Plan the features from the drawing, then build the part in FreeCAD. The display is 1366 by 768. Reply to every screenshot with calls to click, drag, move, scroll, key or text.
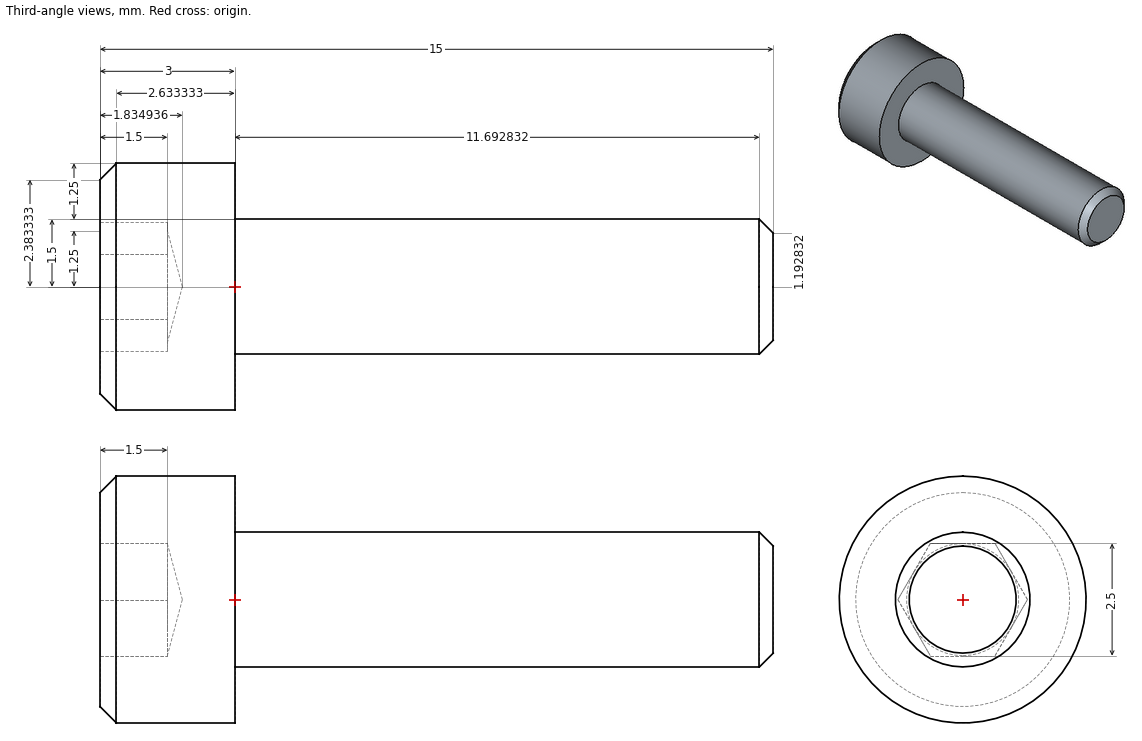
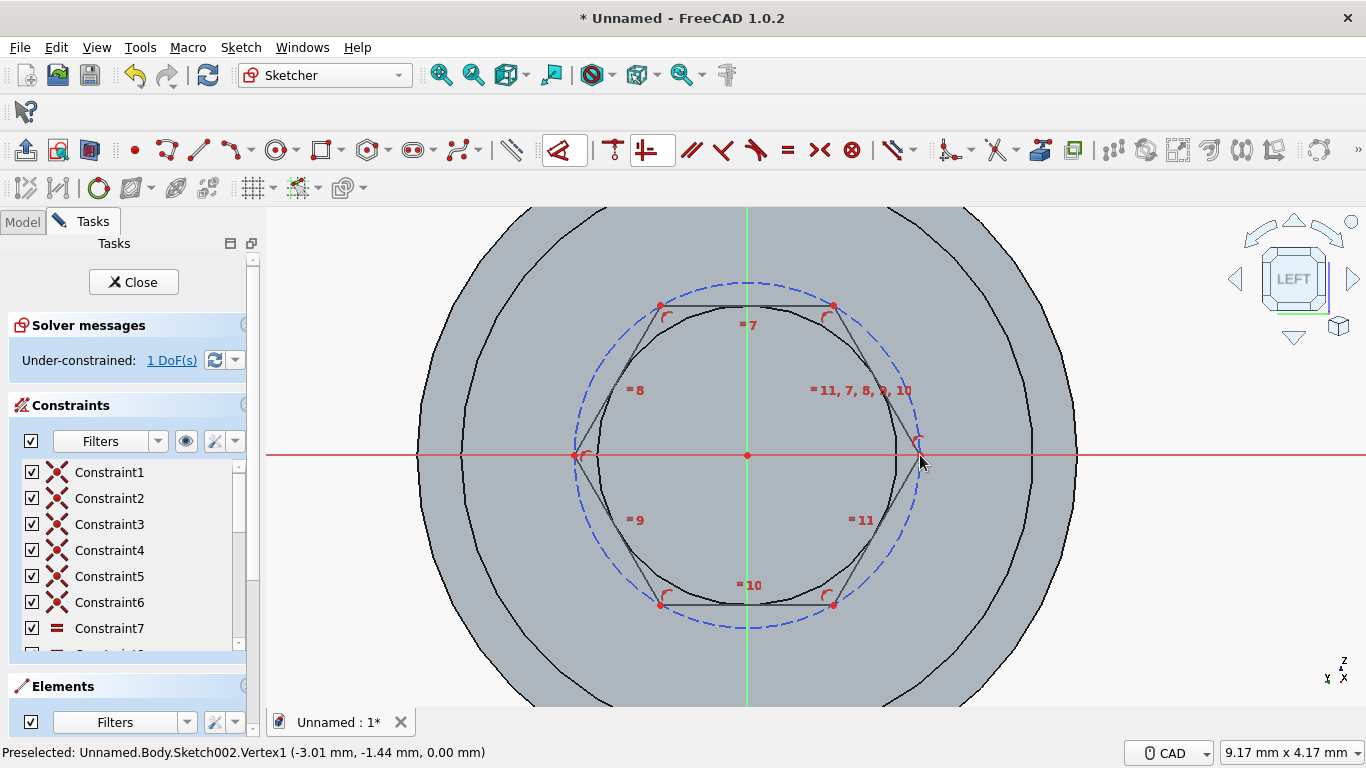
click(661, 605)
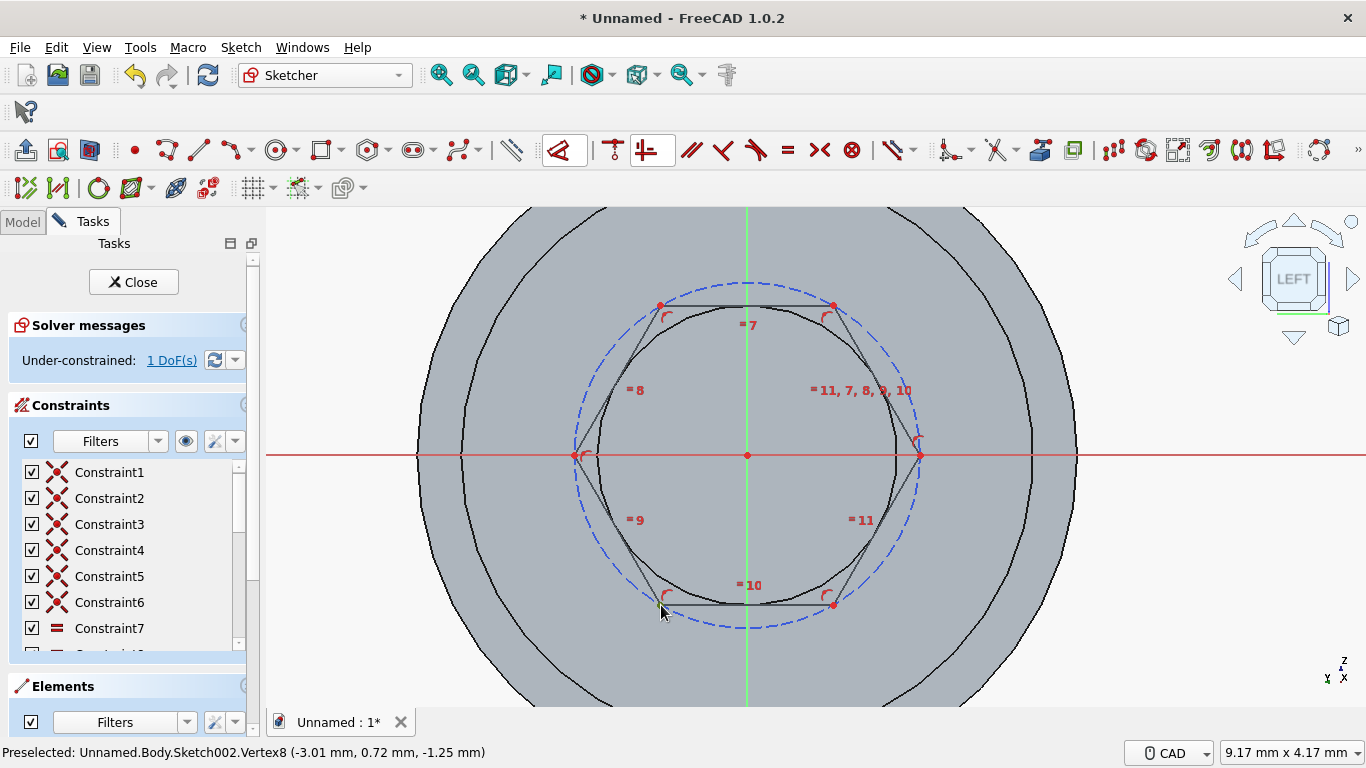
click(834, 306)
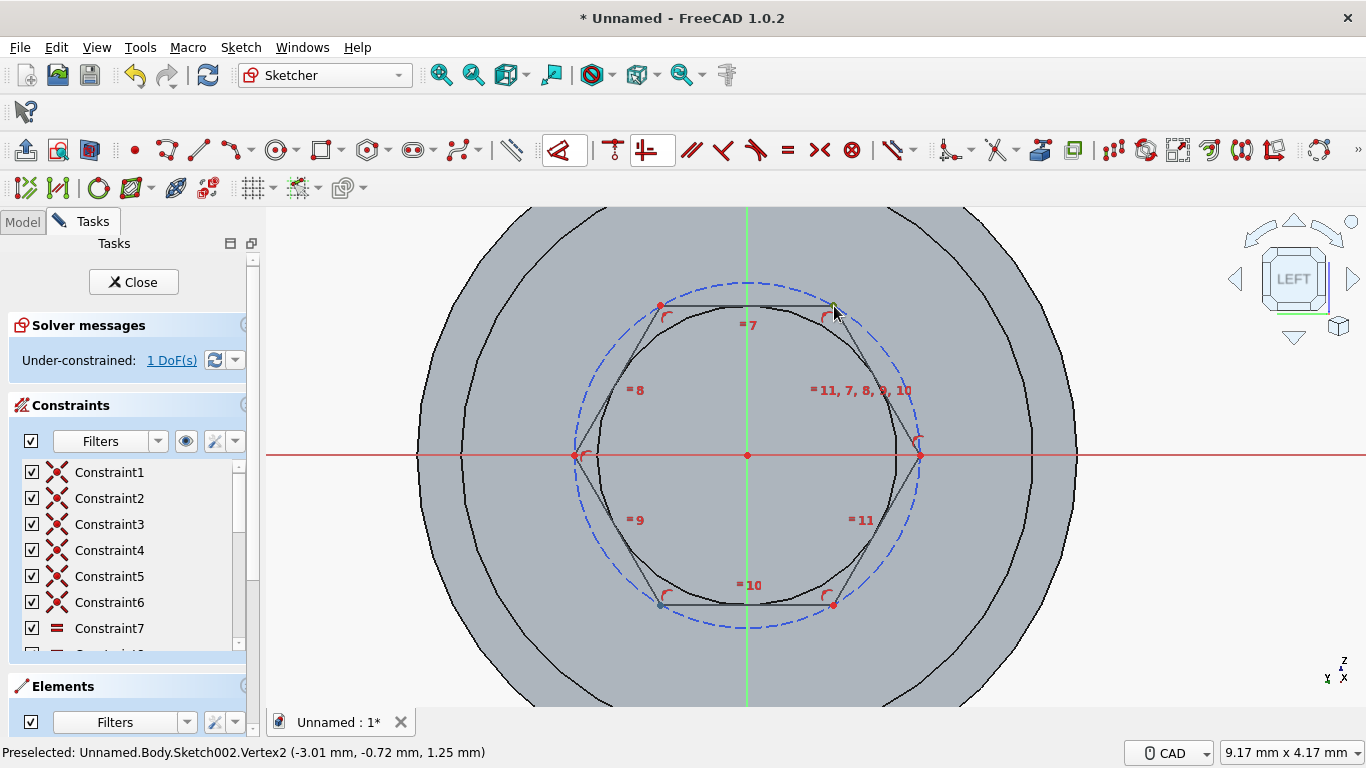
key(i)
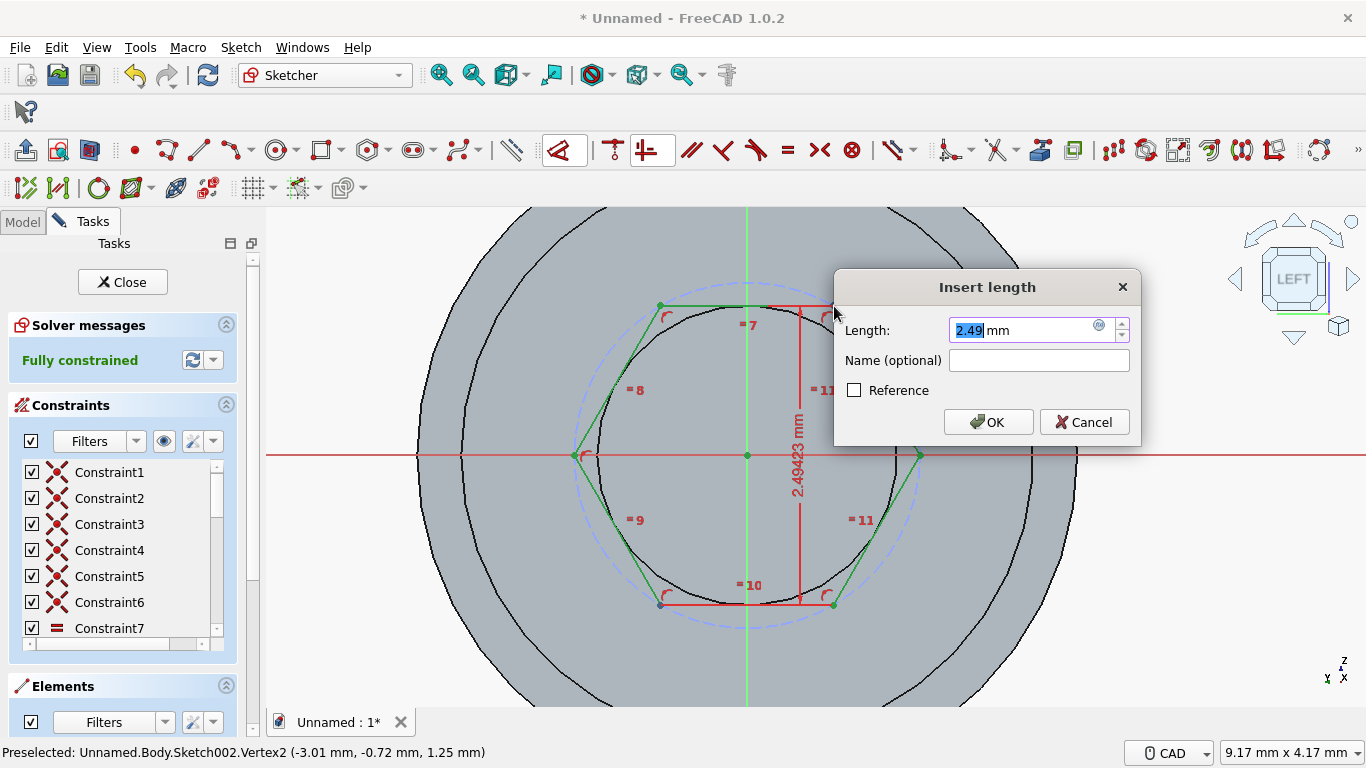
text(2.5)
key(Return)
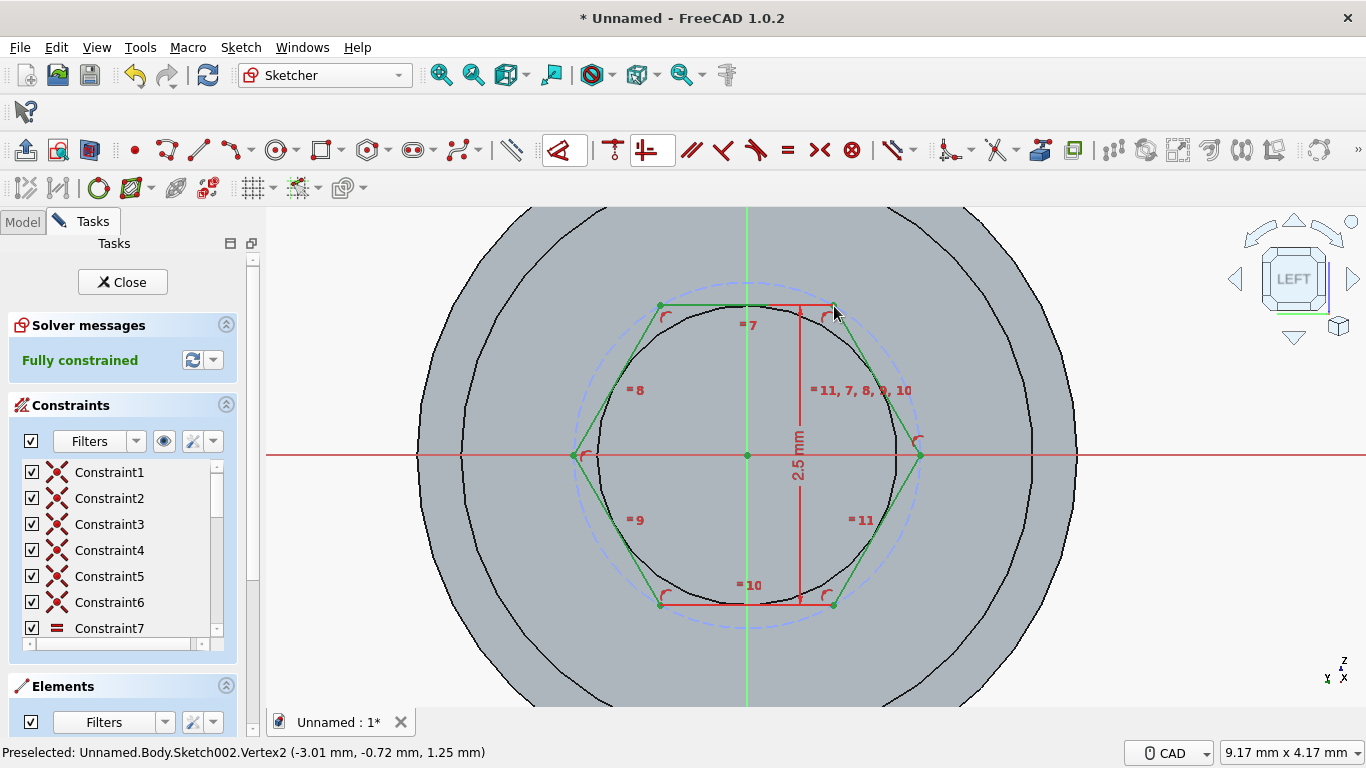
click(123, 282)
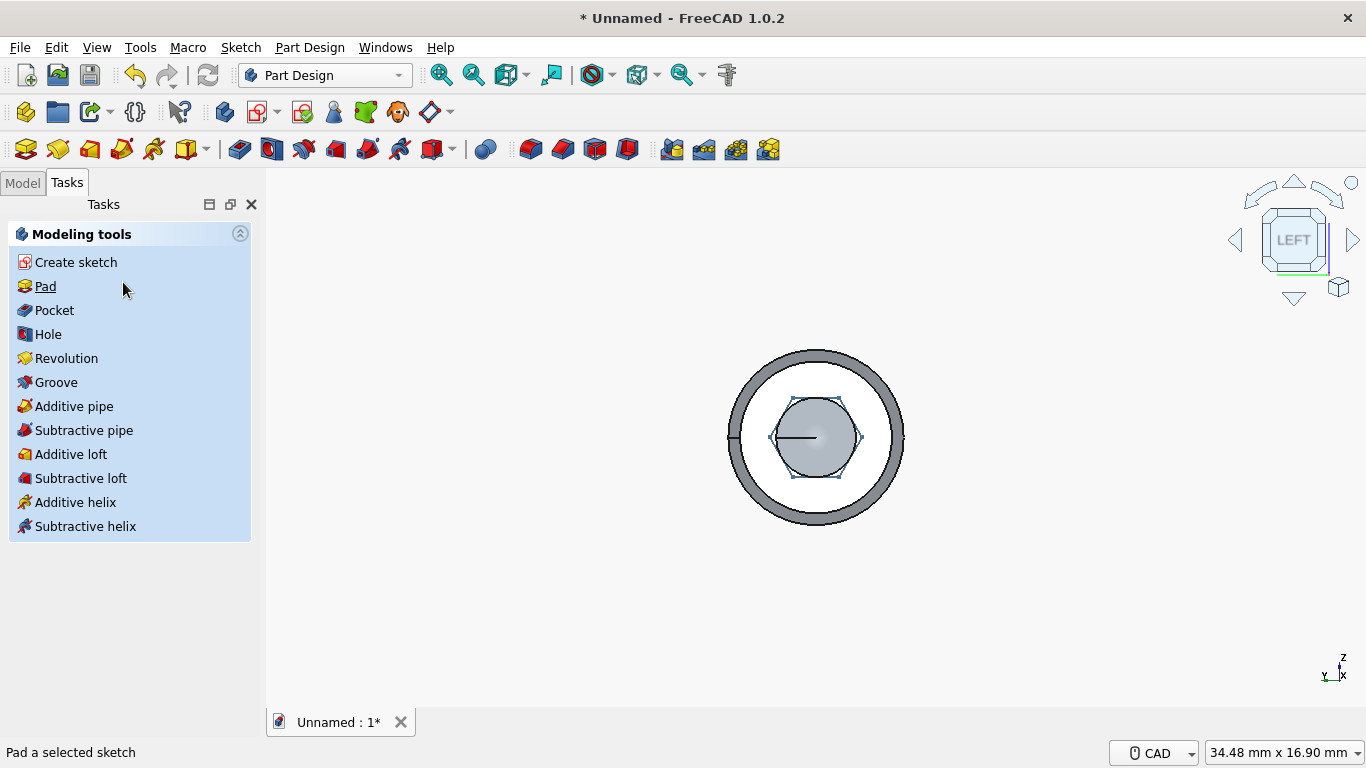
click(240, 150)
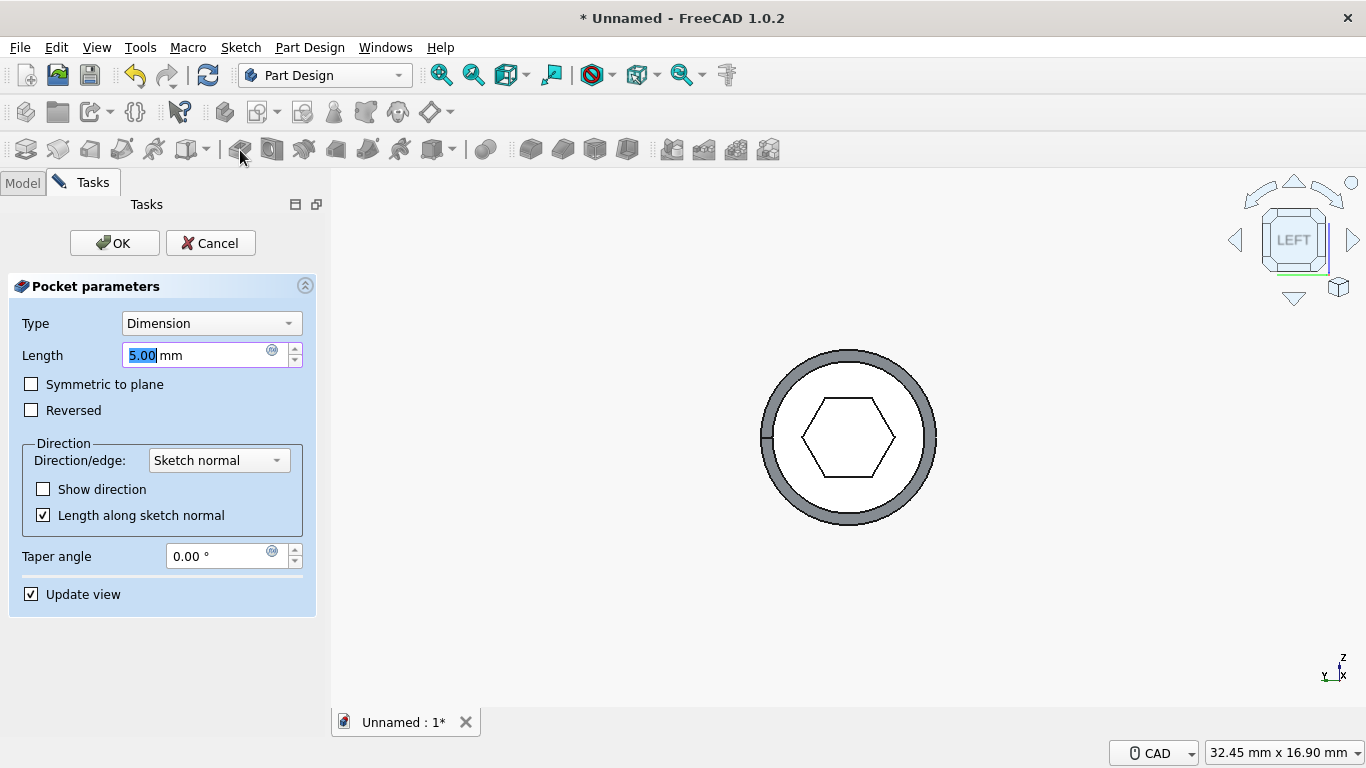
text(1.5)
key(Tab)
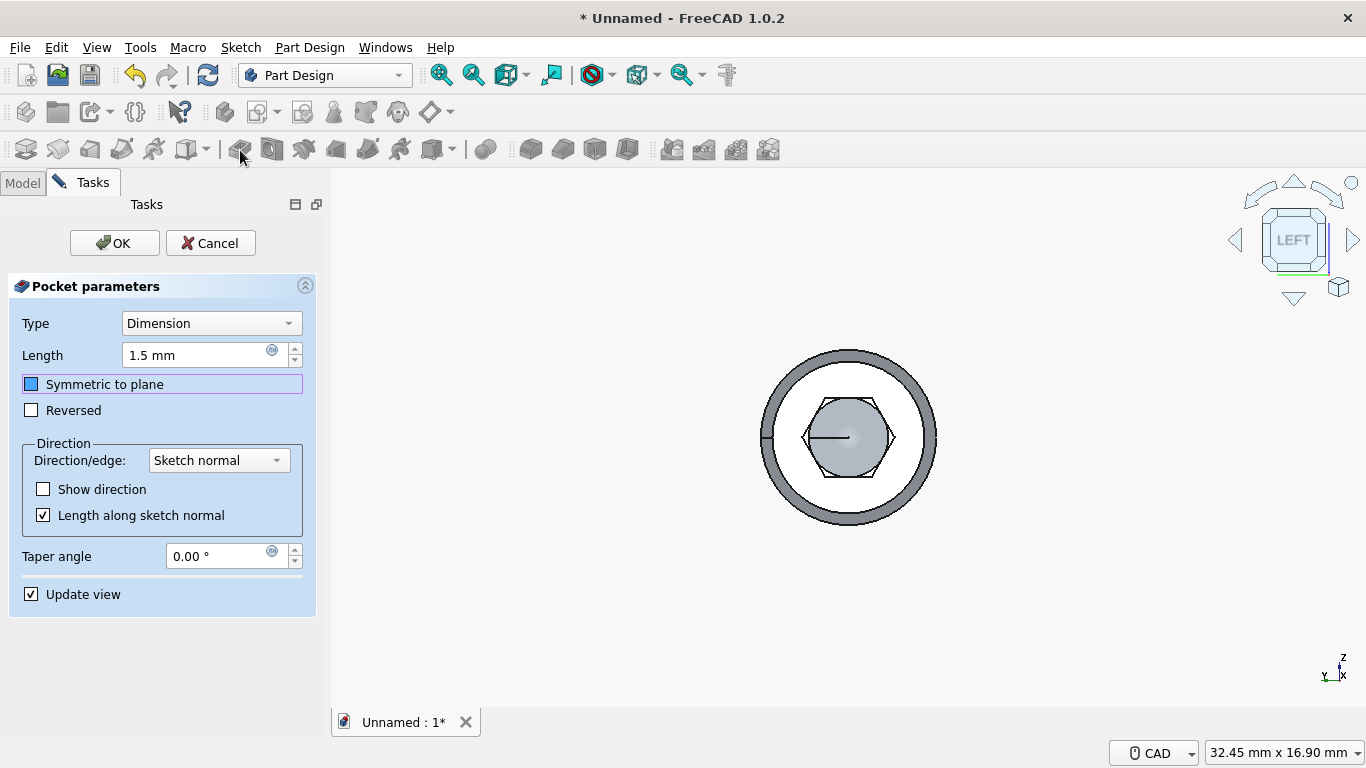
click(115, 243)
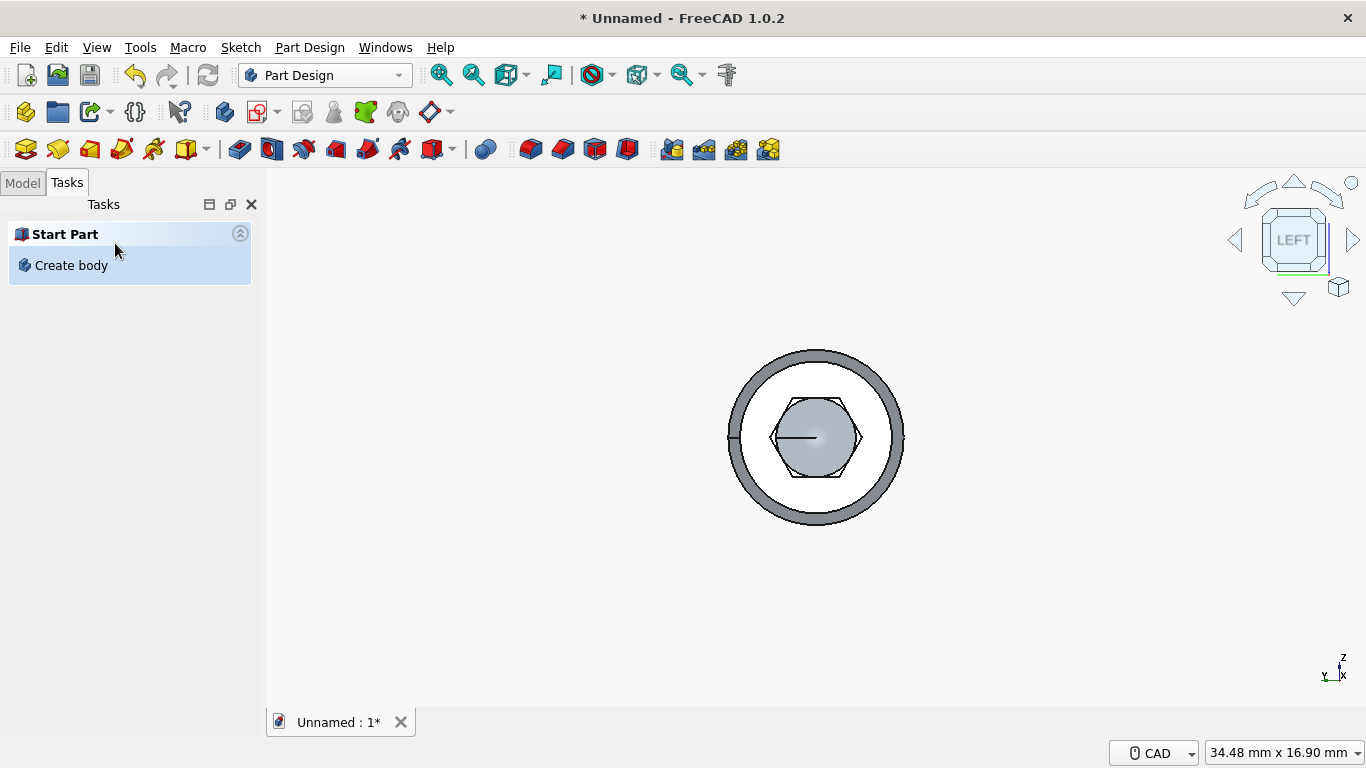
key(0)